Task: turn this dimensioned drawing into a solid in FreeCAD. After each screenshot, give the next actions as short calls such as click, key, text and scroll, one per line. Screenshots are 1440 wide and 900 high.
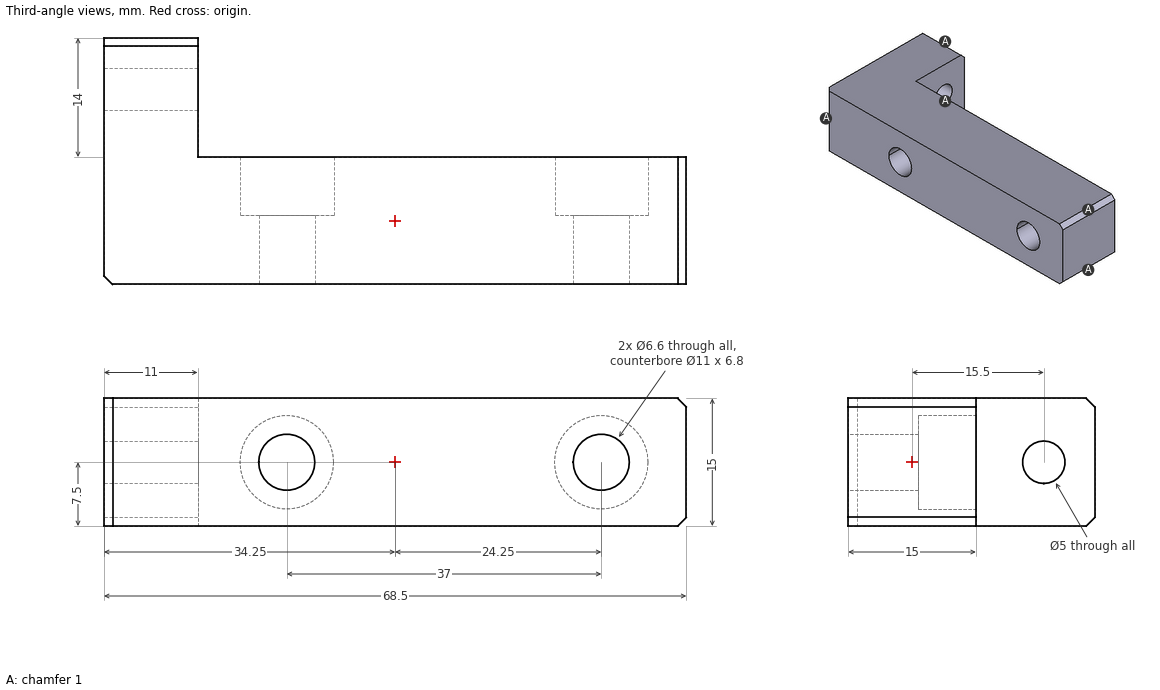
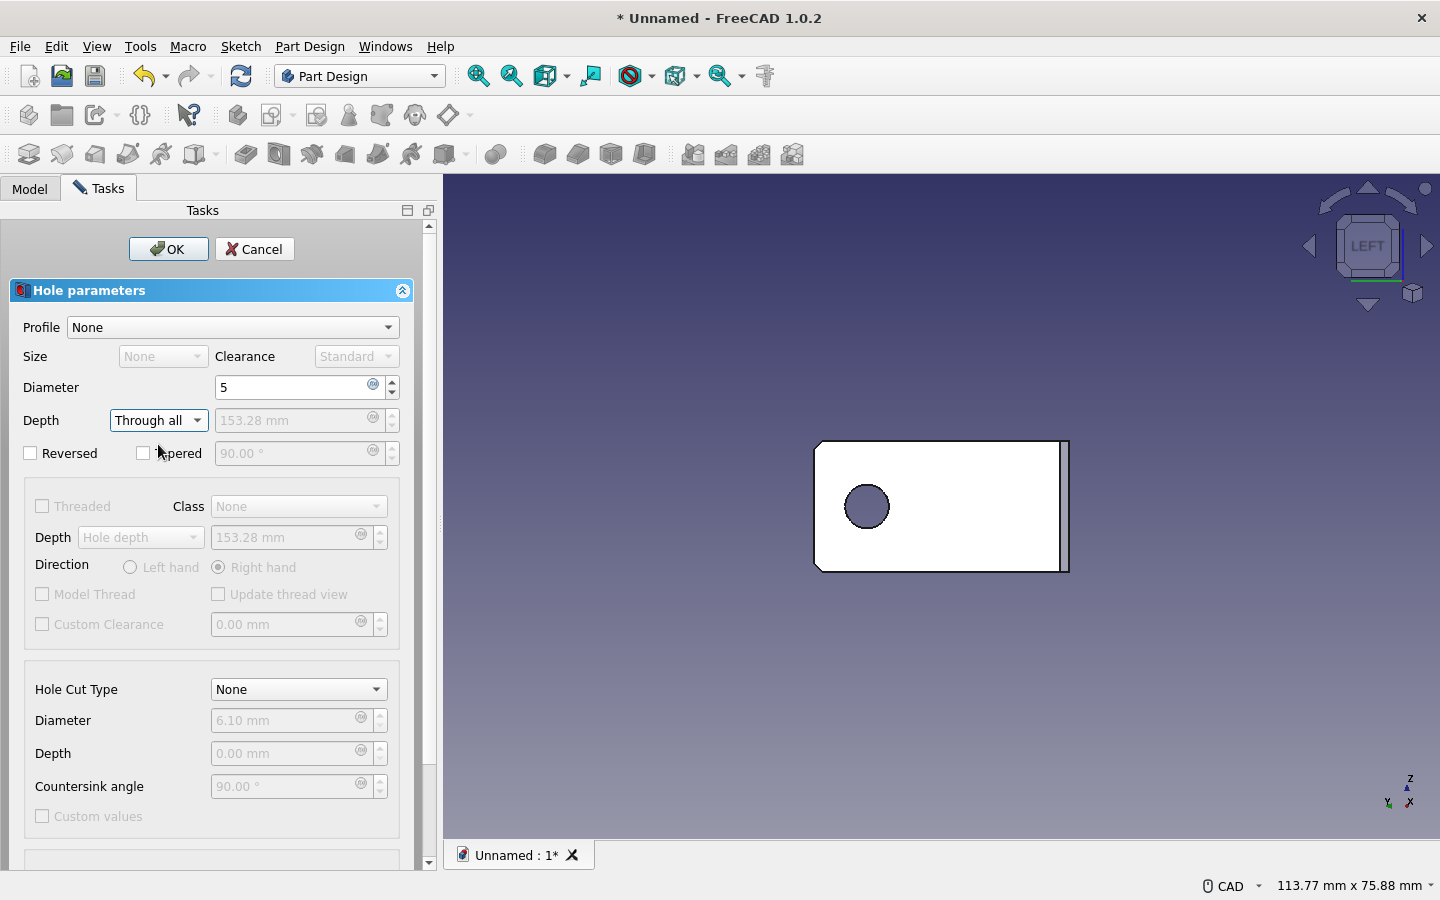
click(169, 249)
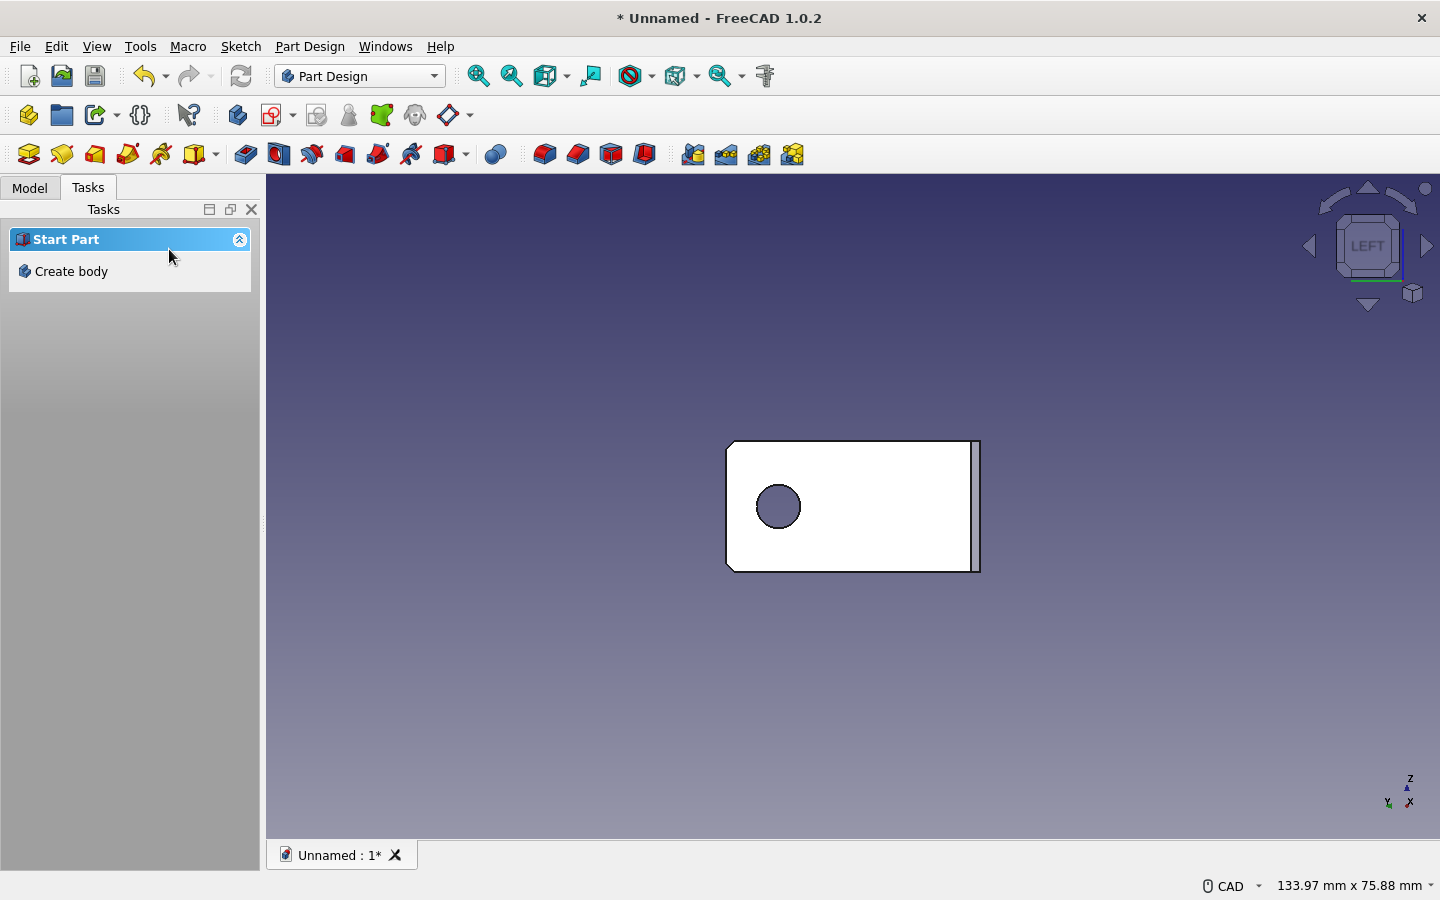
key(0)